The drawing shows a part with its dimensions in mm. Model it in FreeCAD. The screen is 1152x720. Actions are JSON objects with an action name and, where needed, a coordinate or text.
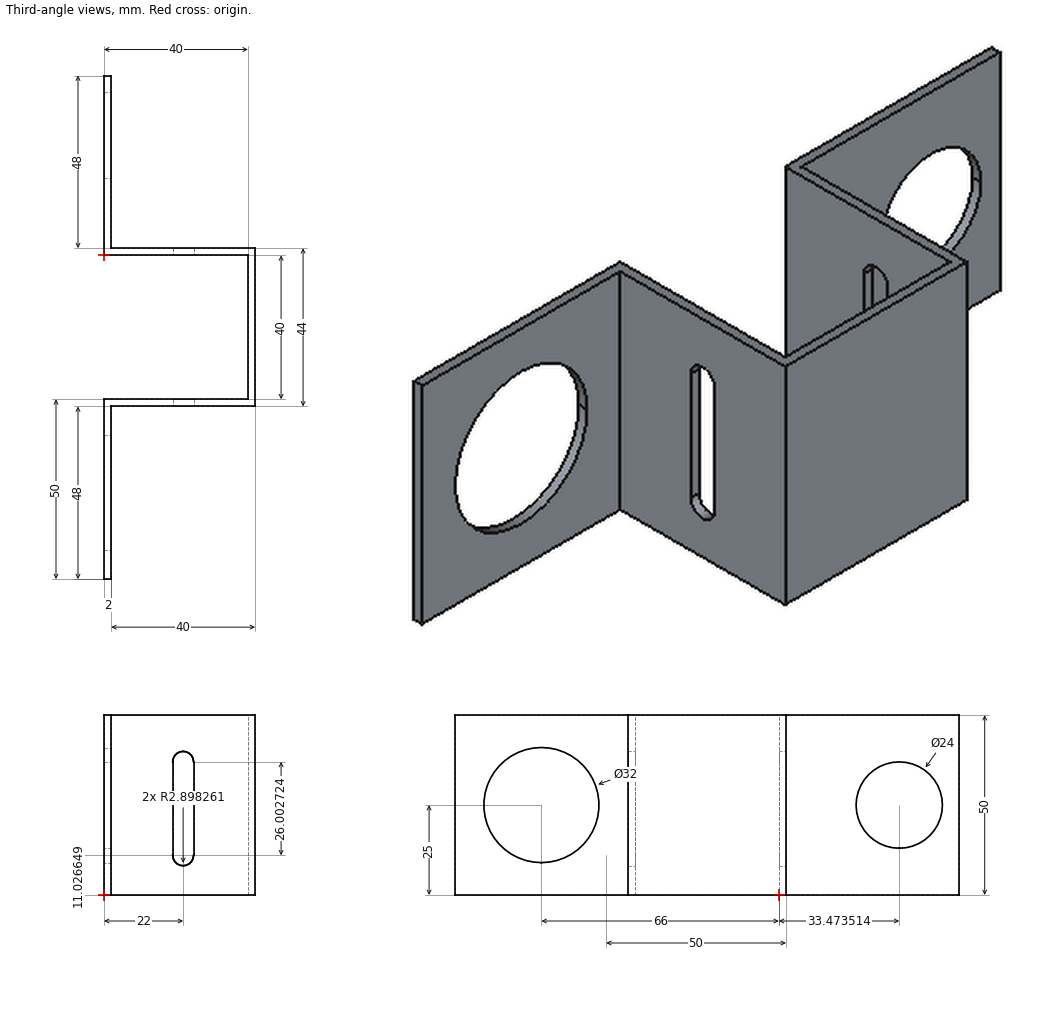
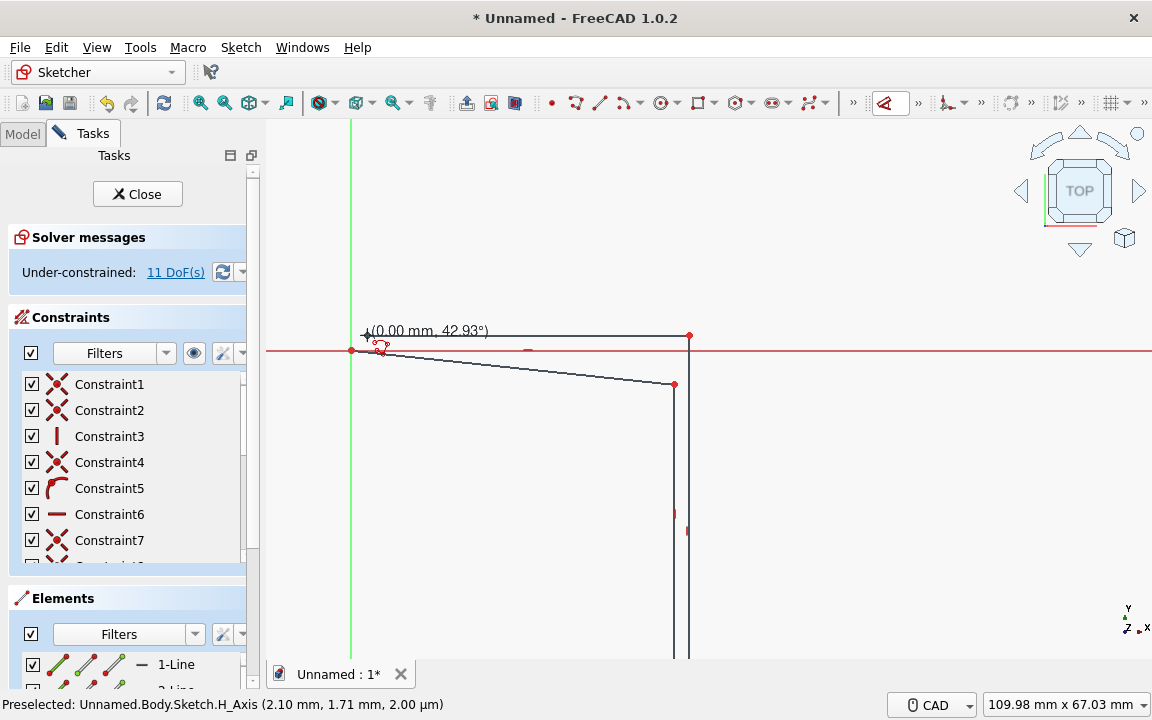
{"action": "scroll", "coordinate": [692, 336], "scroll_direction": "down", "scroll_amount": 6}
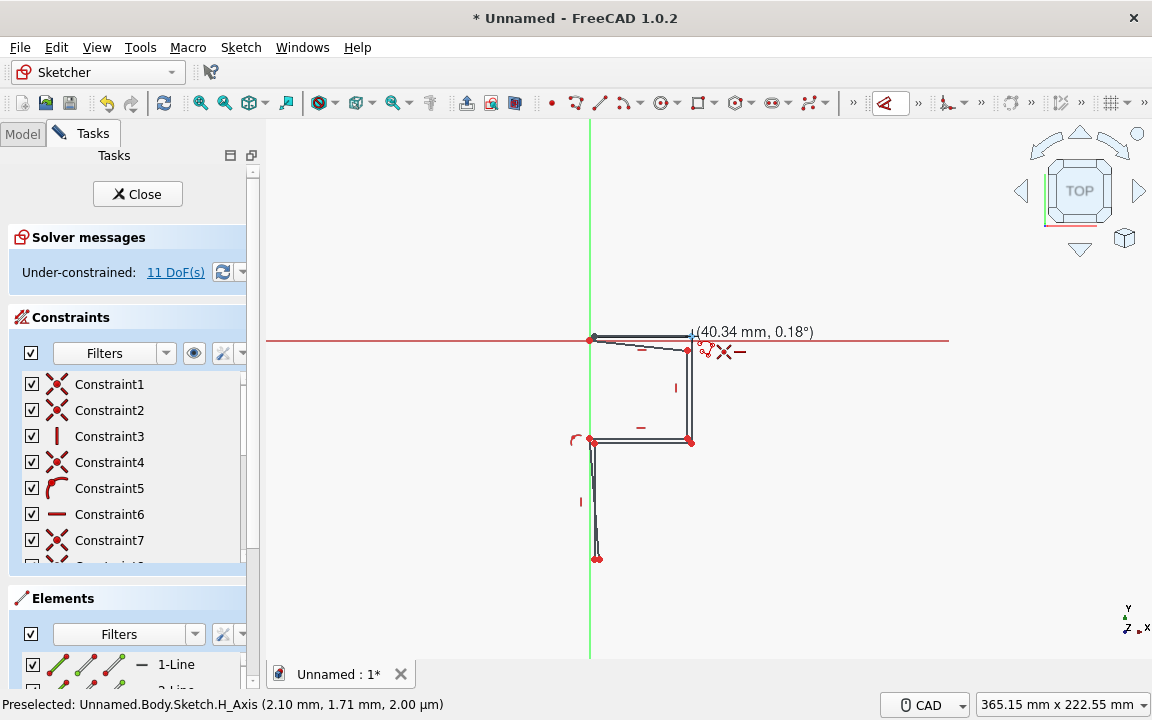
{"action": "scroll", "coordinate": [594, 219], "scroll_direction": "up", "scroll_amount": 6}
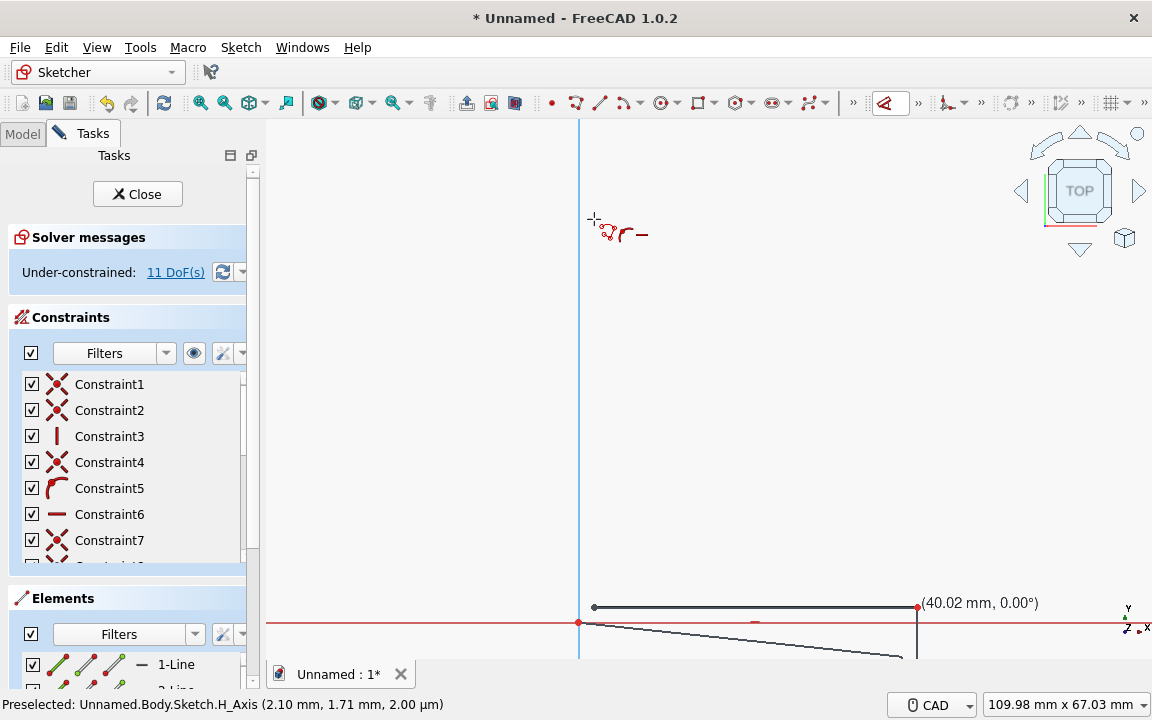
{"action": "left_click", "coordinate": [595, 220]}
{"action": "left_click", "coordinate": [588, 220]}
{"action": "left_click", "coordinate": [579, 623]}
{"action": "key", "text": "Escape"}
{"action": "key", "text": "Escape"}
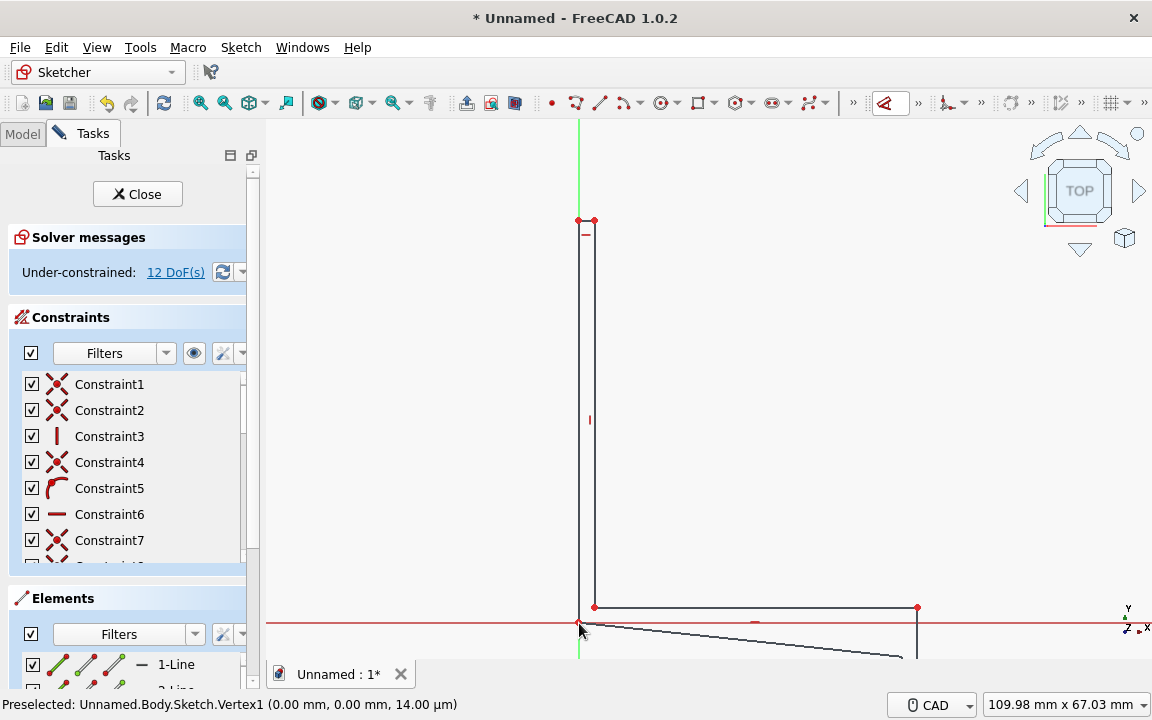
{"action": "scroll", "coordinate": [594, 219], "scroll_direction": "down", "scroll_amount": 6}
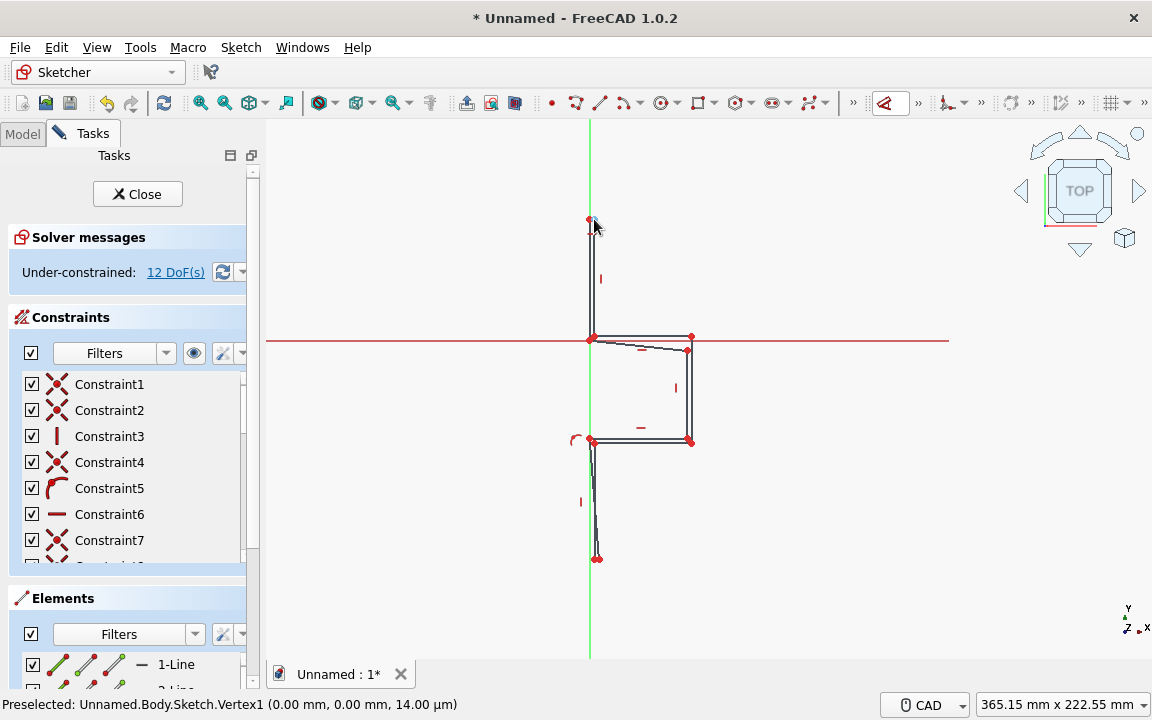
{"action": "scroll", "coordinate": [619, 344], "scroll_direction": "up", "scroll_amount": 8}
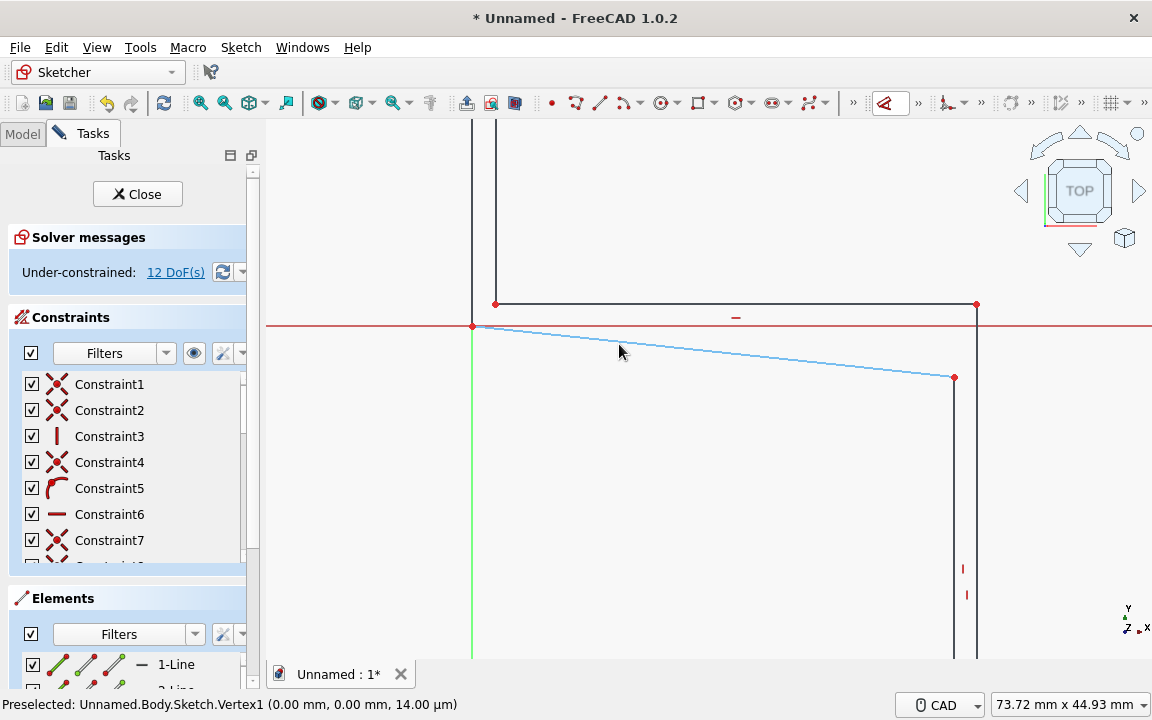
{"action": "left_click", "coordinate": [617, 341]}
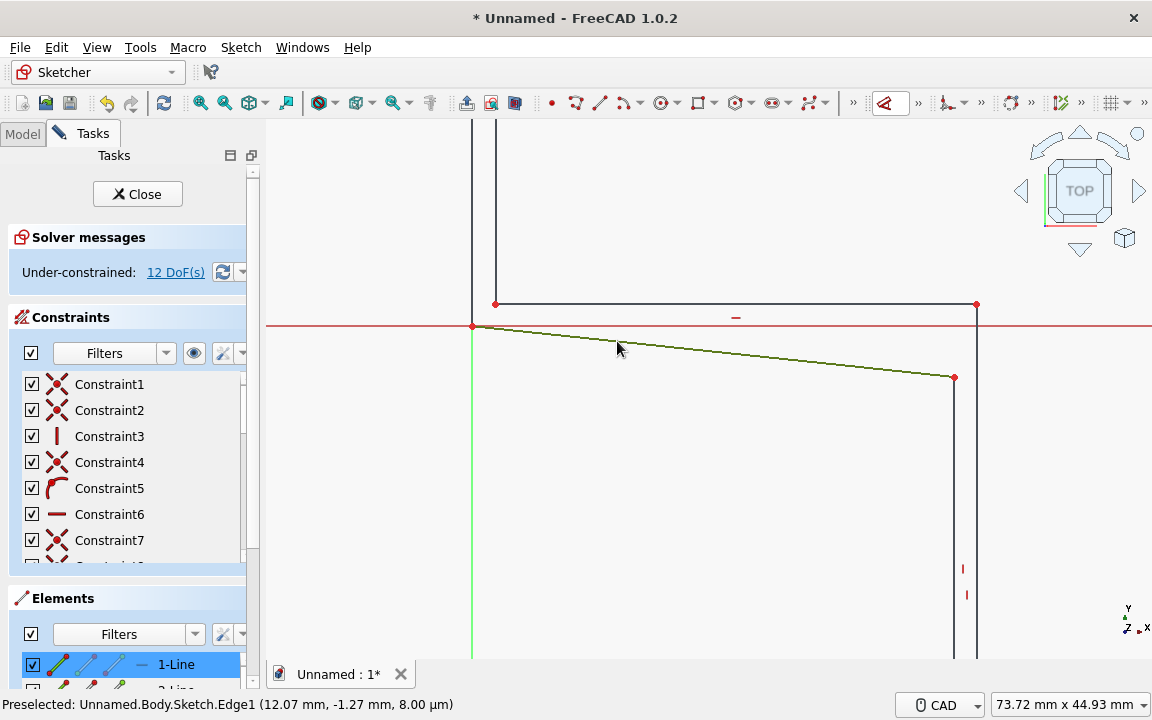
{"action": "key", "text": "h"}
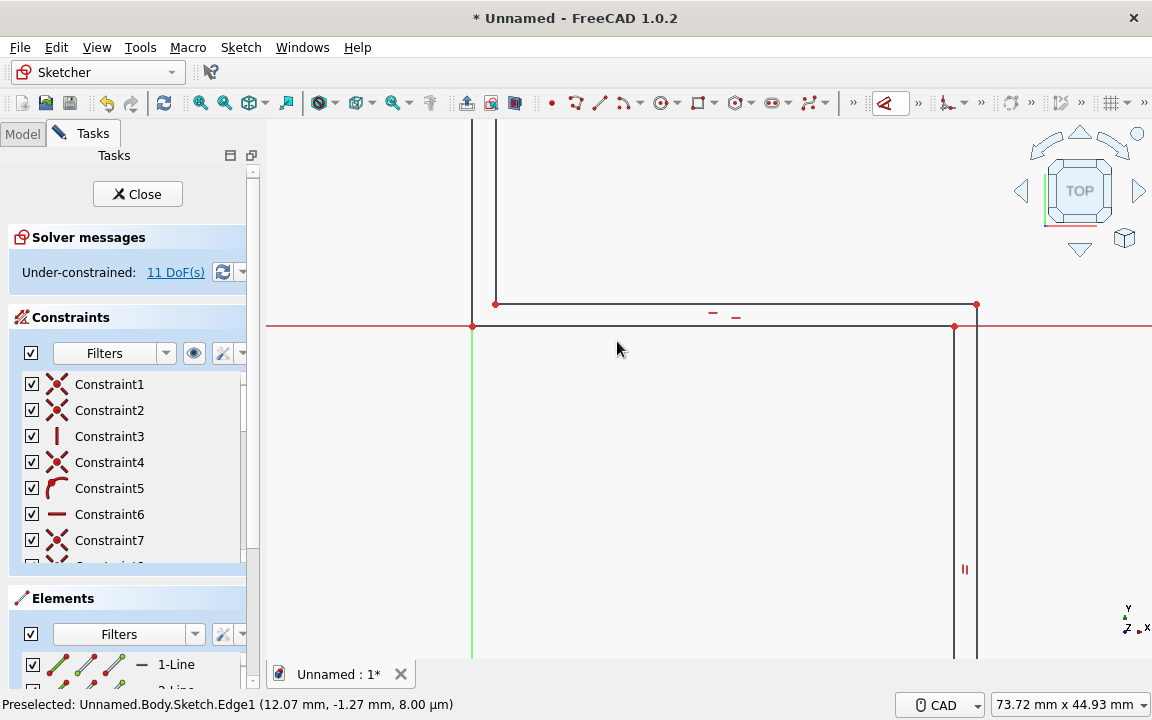
{"action": "scroll", "coordinate": [619, 344], "scroll_direction": "down", "scroll_amount": 8}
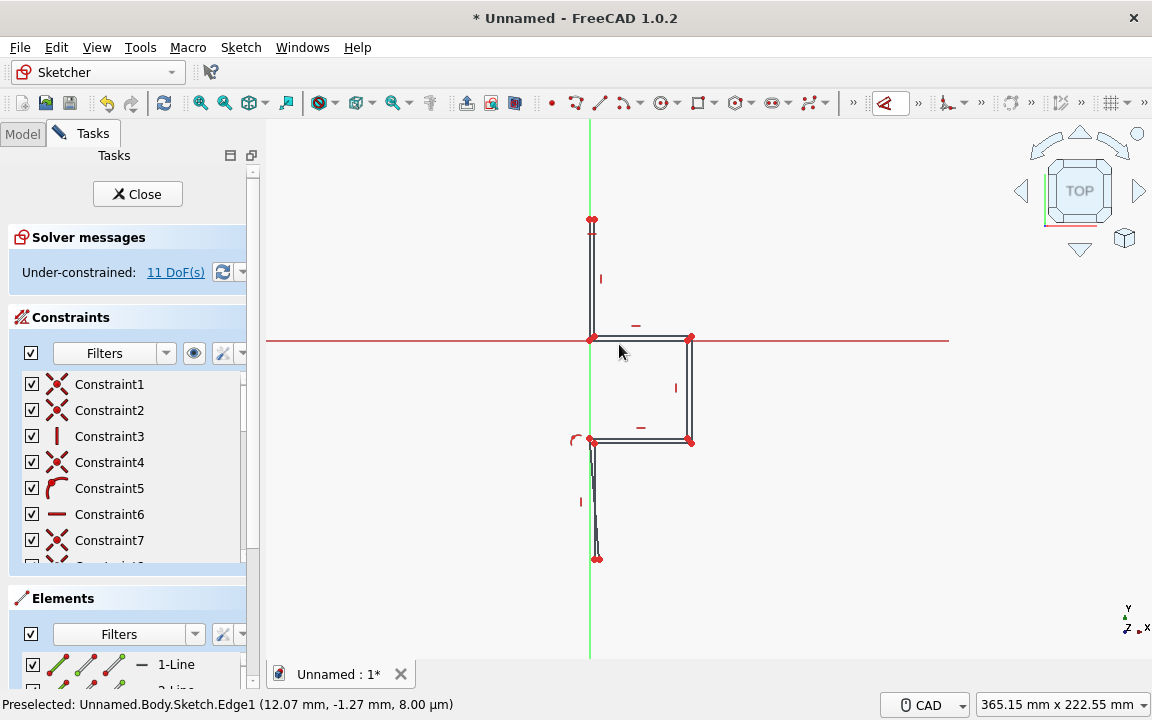
{"action": "scroll", "coordinate": [592, 475], "scroll_direction": "up", "scroll_amount": 10}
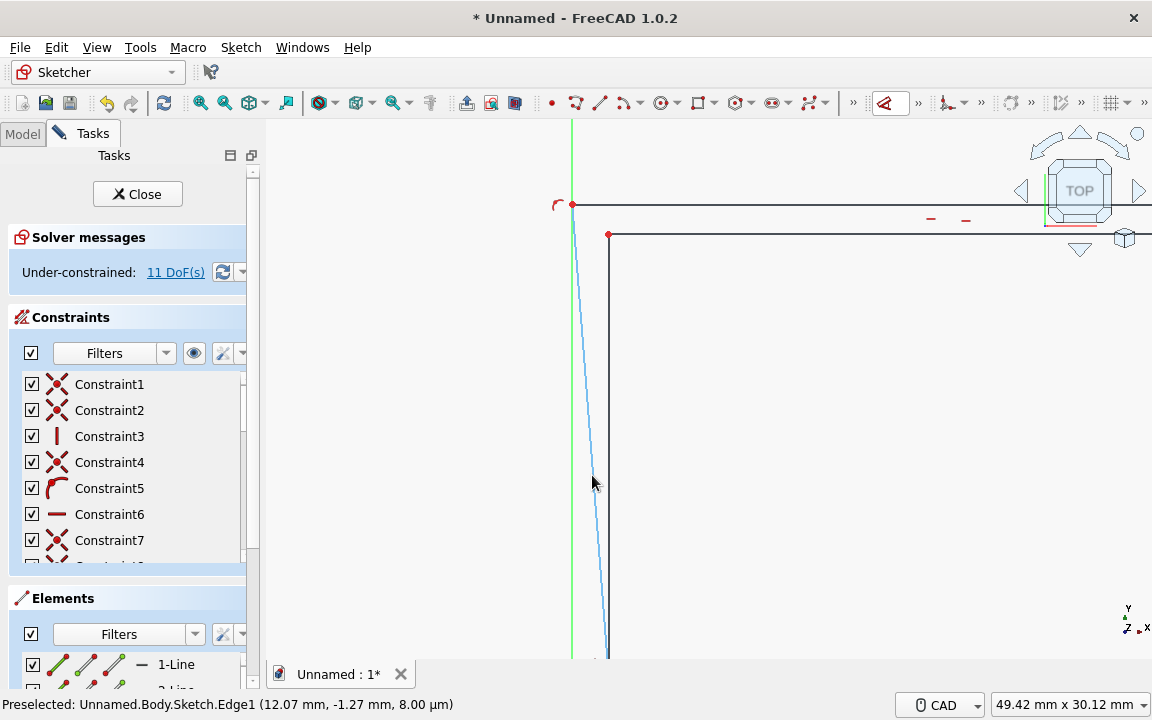
{"action": "left_click", "coordinate": [593, 473]}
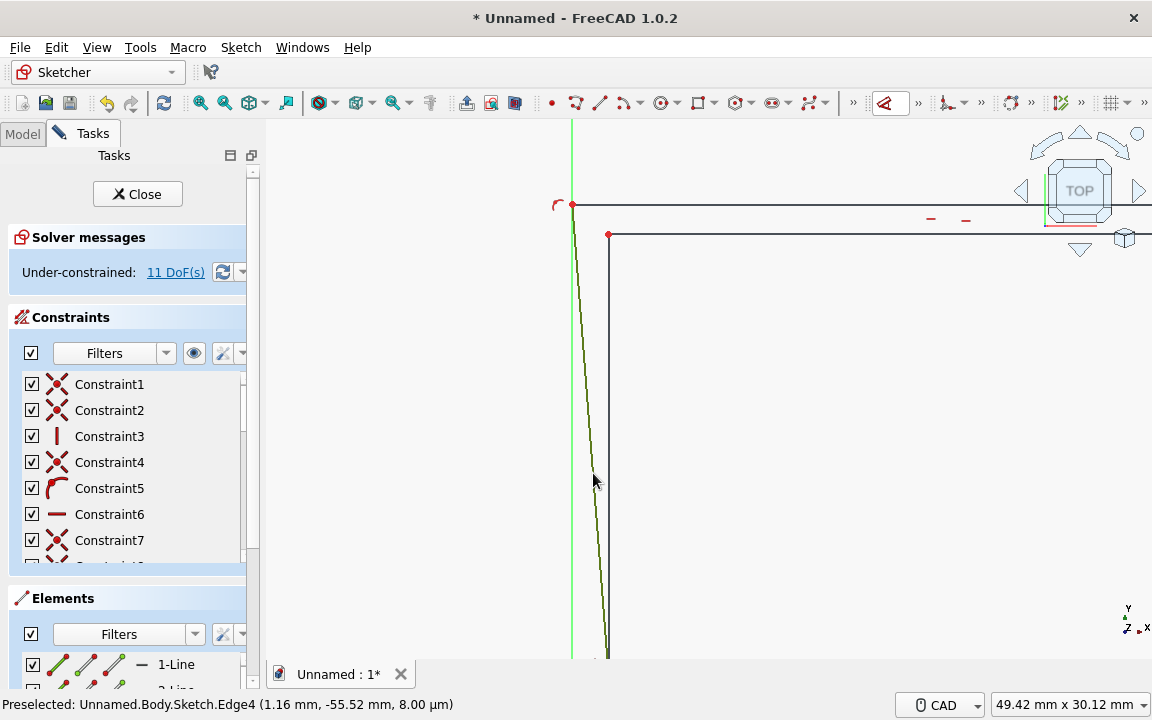
{"action": "key", "text": "v"}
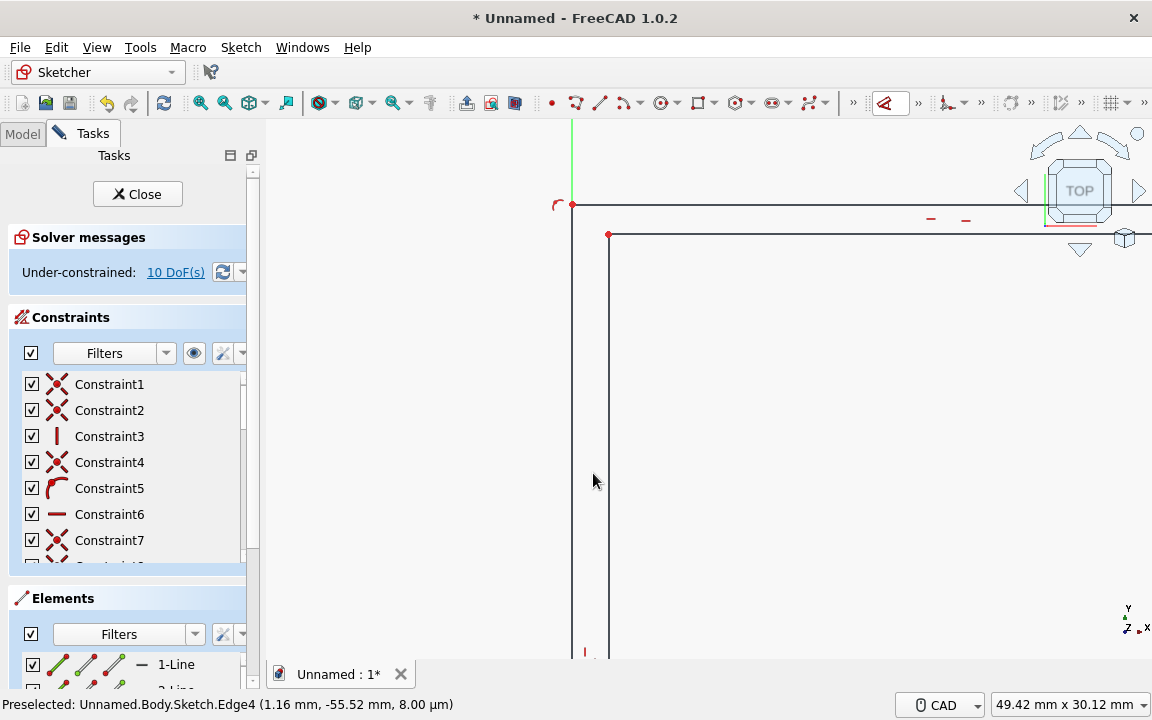
{"action": "scroll", "coordinate": [592, 475], "scroll_direction": "down", "scroll_amount": 10}